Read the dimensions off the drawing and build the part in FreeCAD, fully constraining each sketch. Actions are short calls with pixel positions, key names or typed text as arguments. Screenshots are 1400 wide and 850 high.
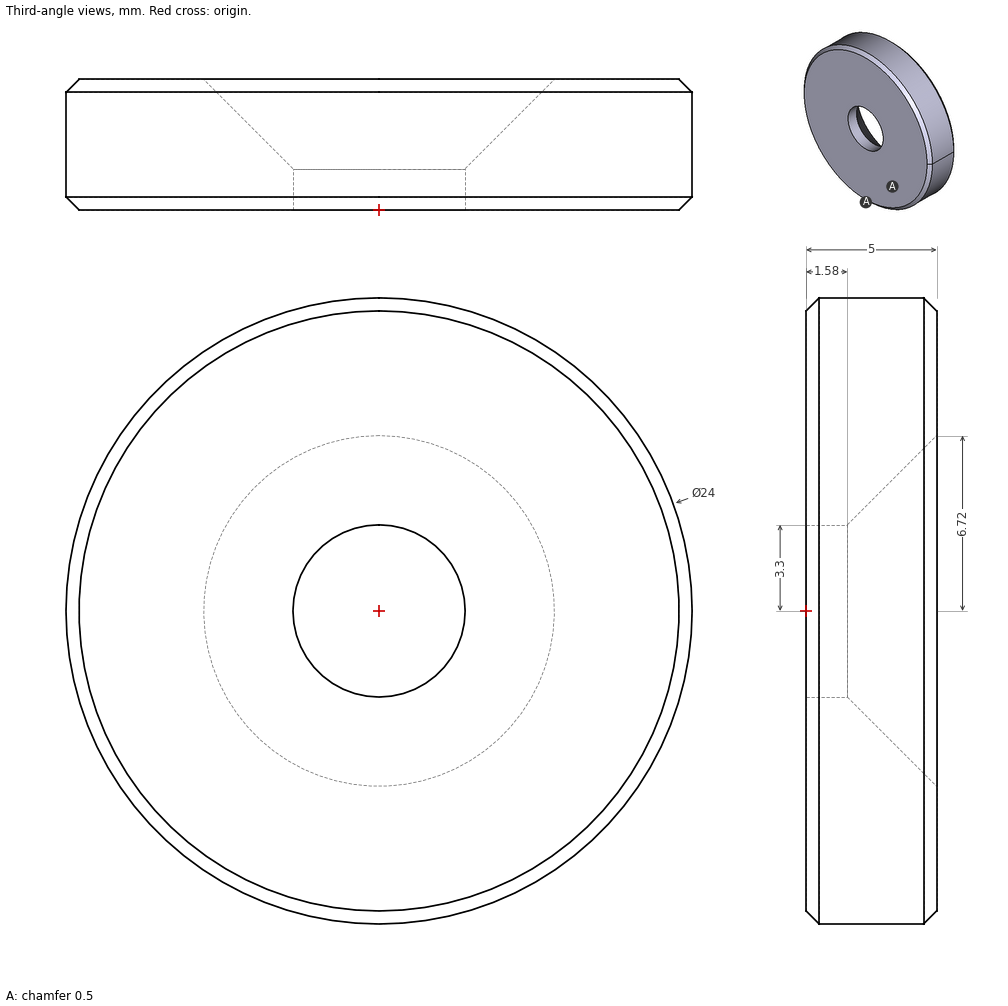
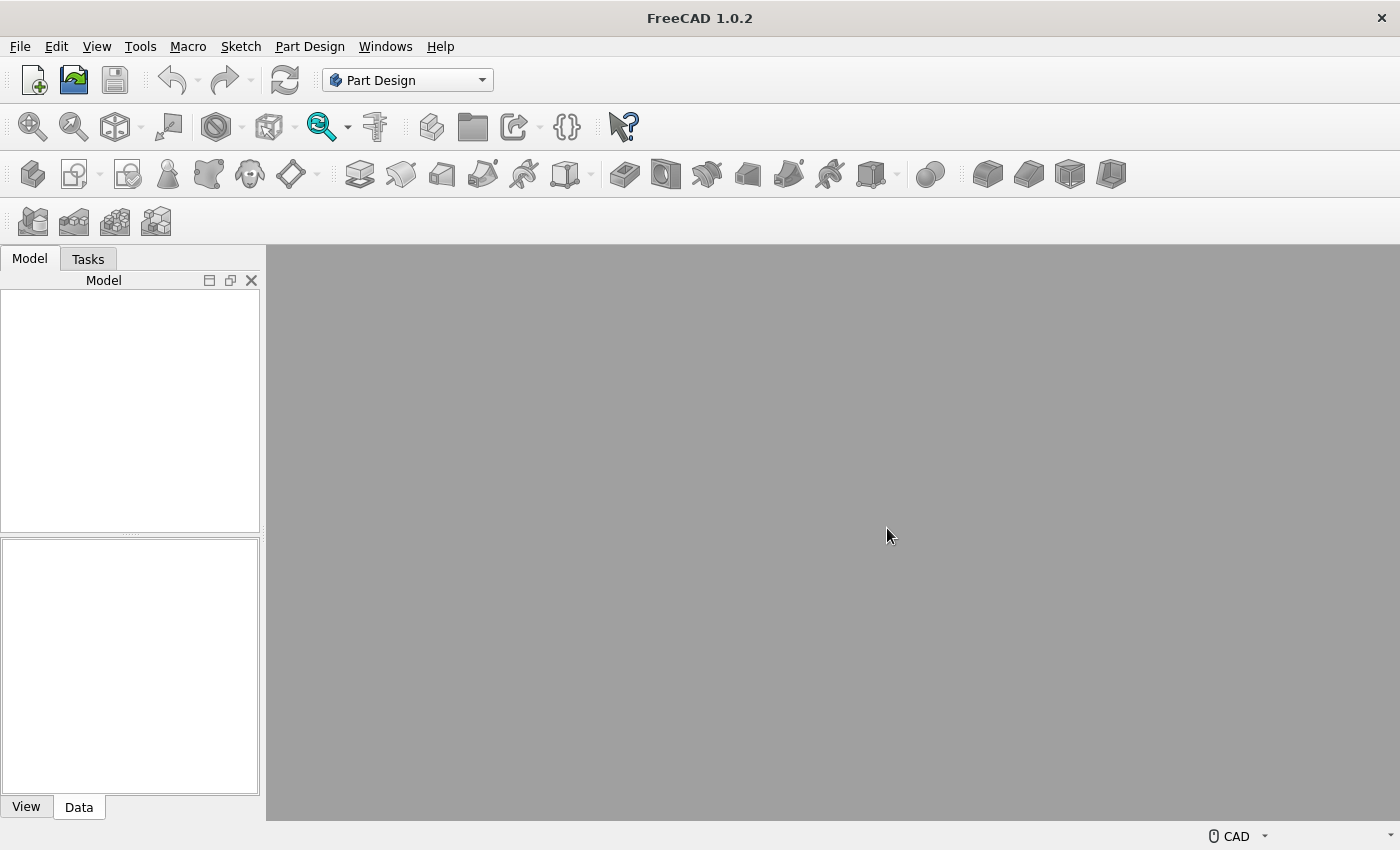
click(33, 80)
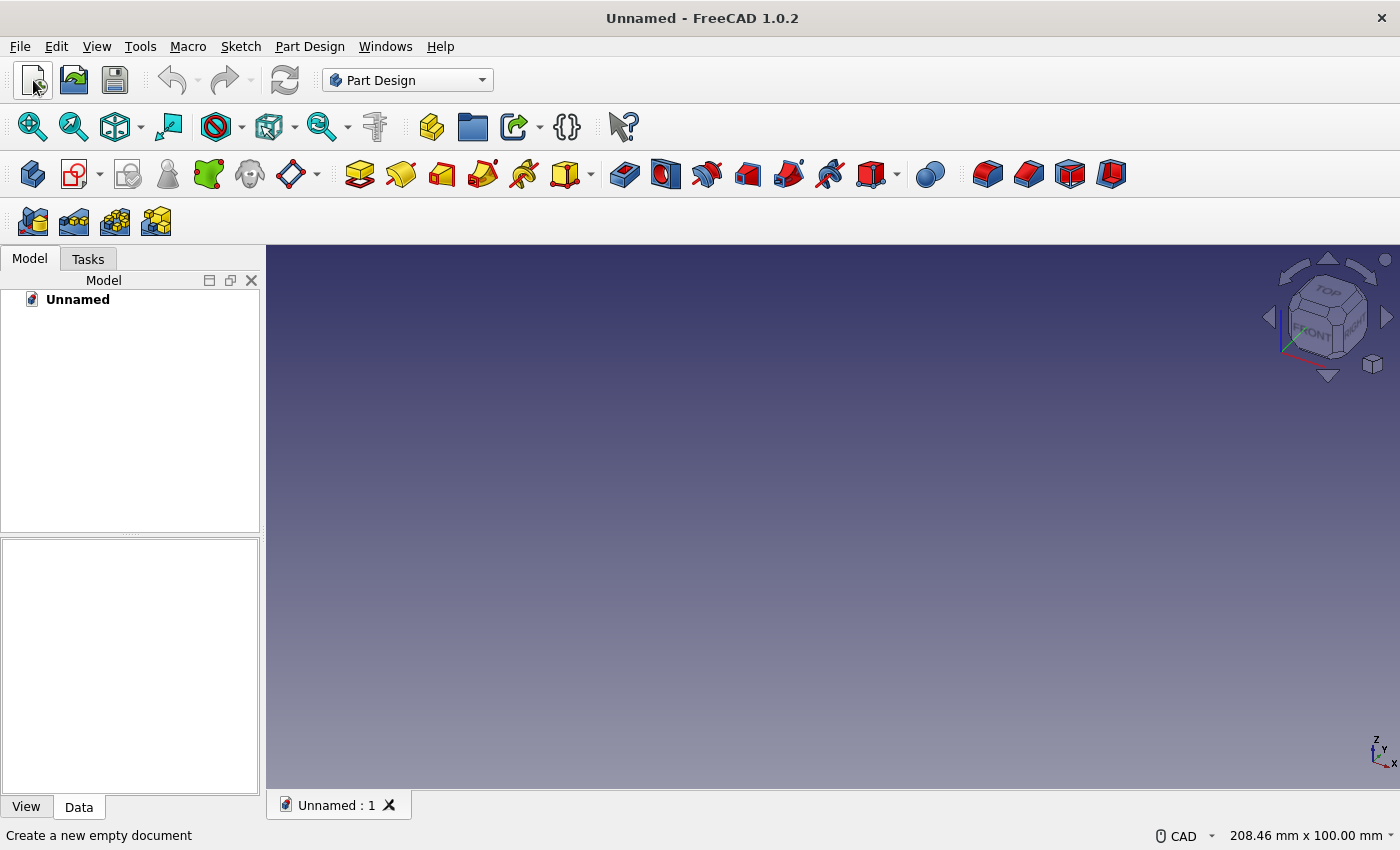
click(74, 174)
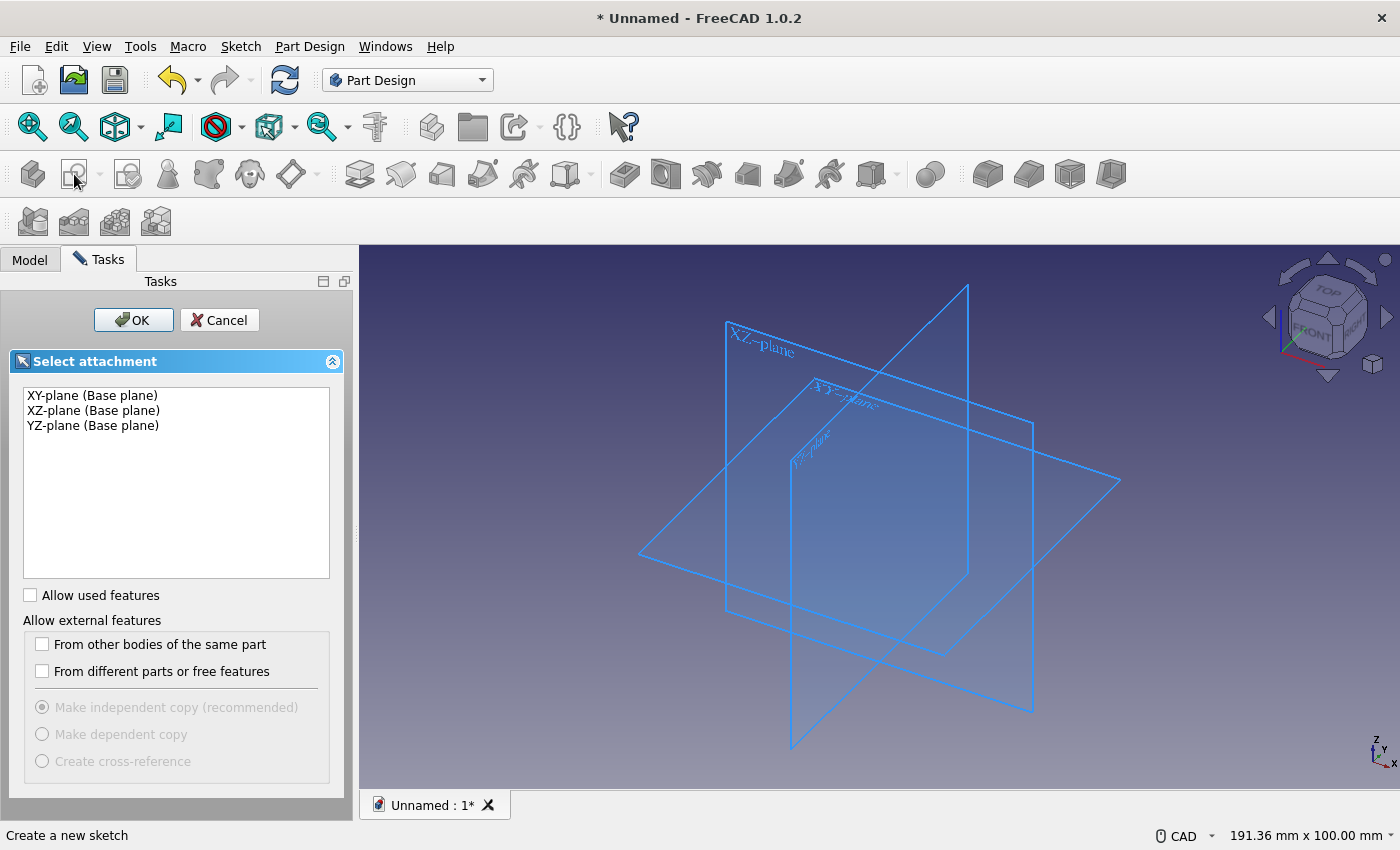
click(84, 410)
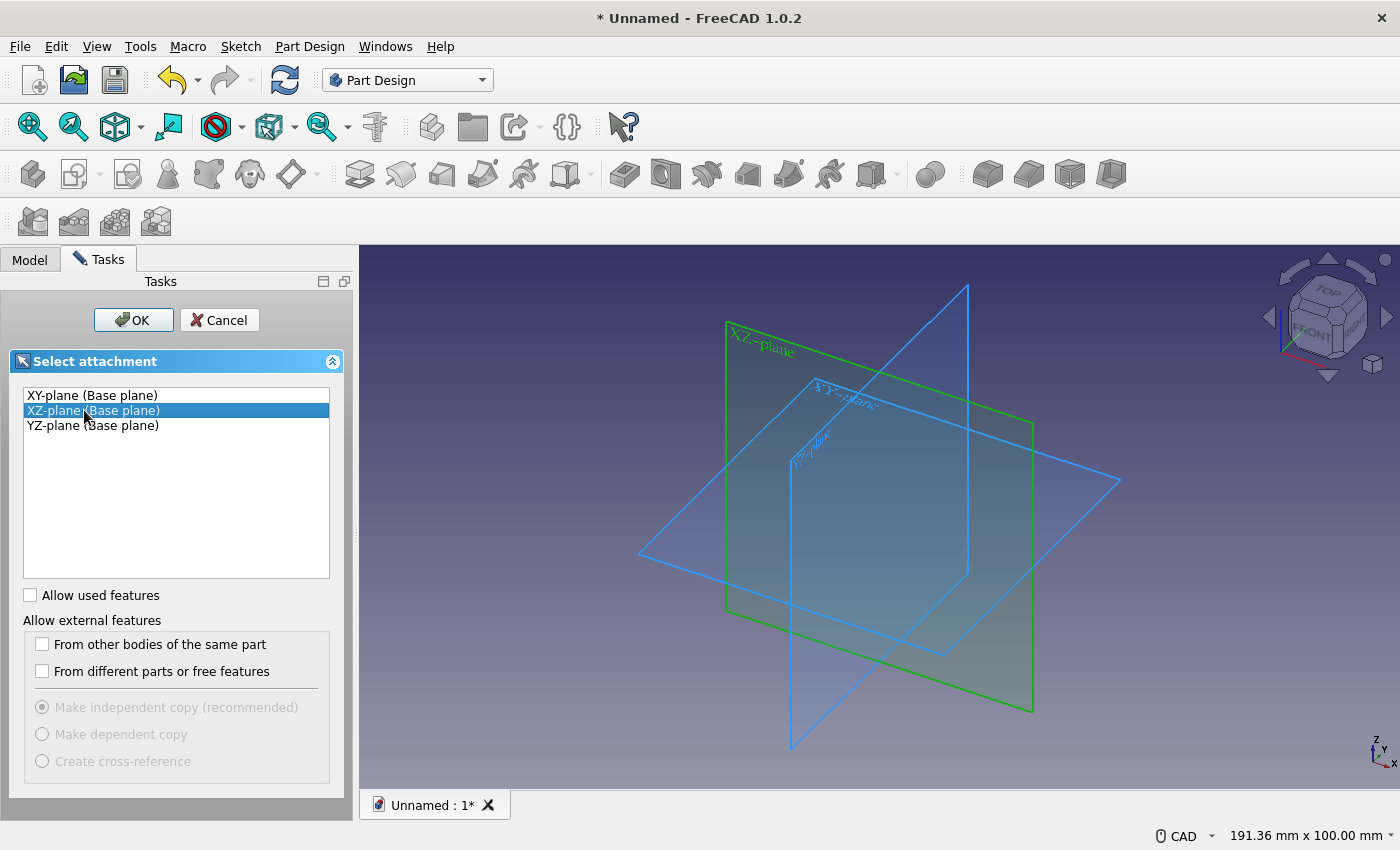
click(134, 320)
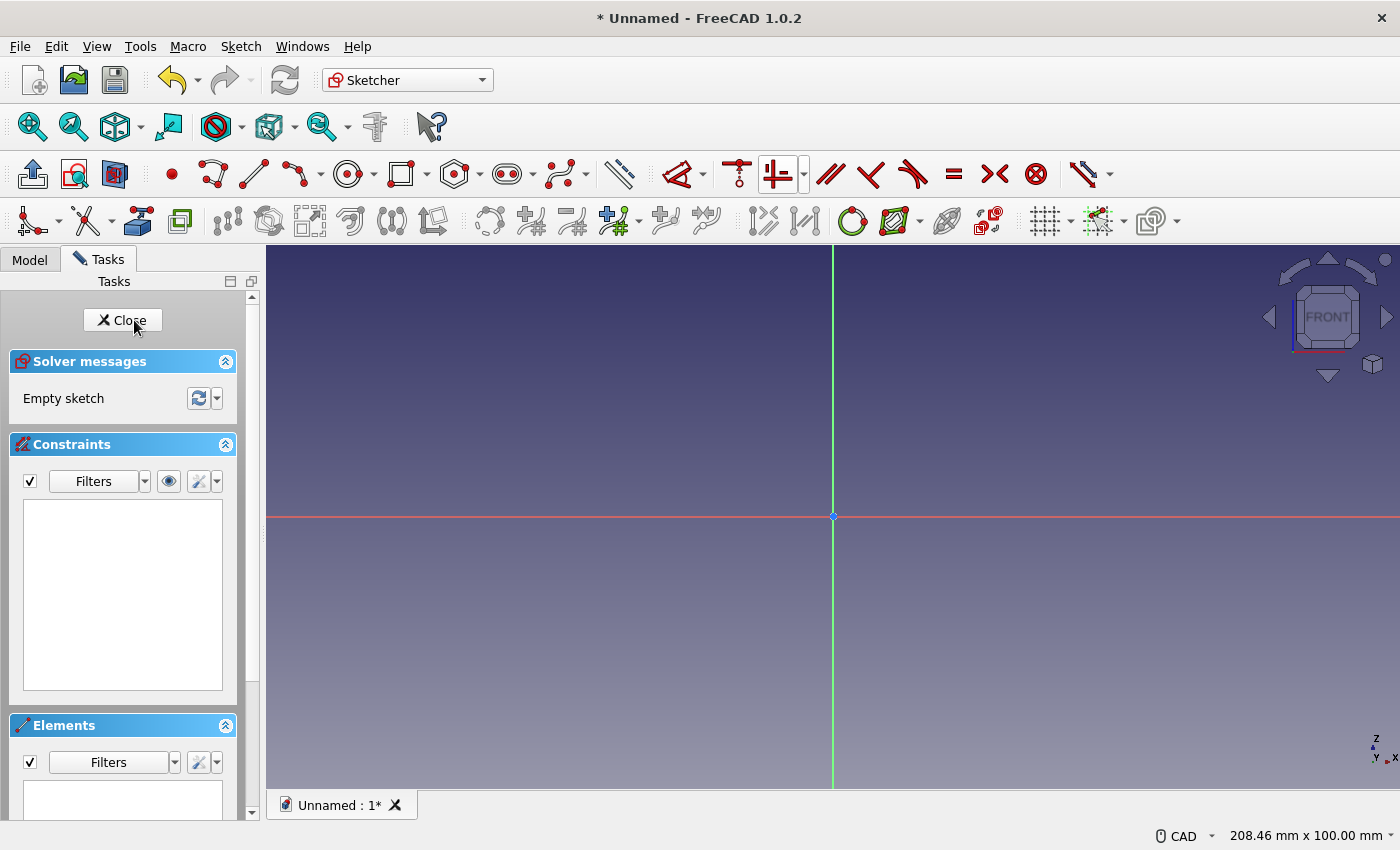
scroll(873, 517, up, 5)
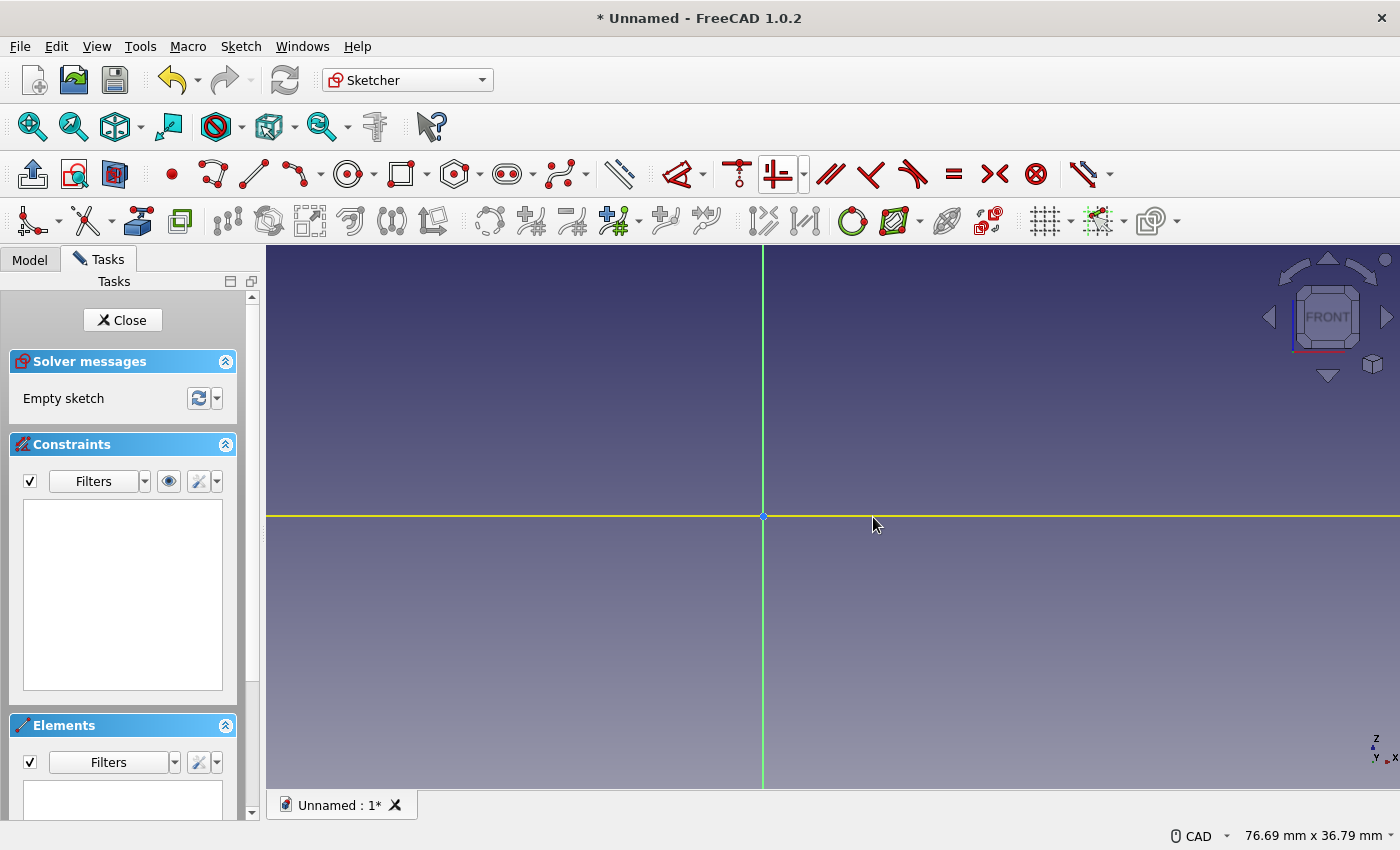
click(348, 174)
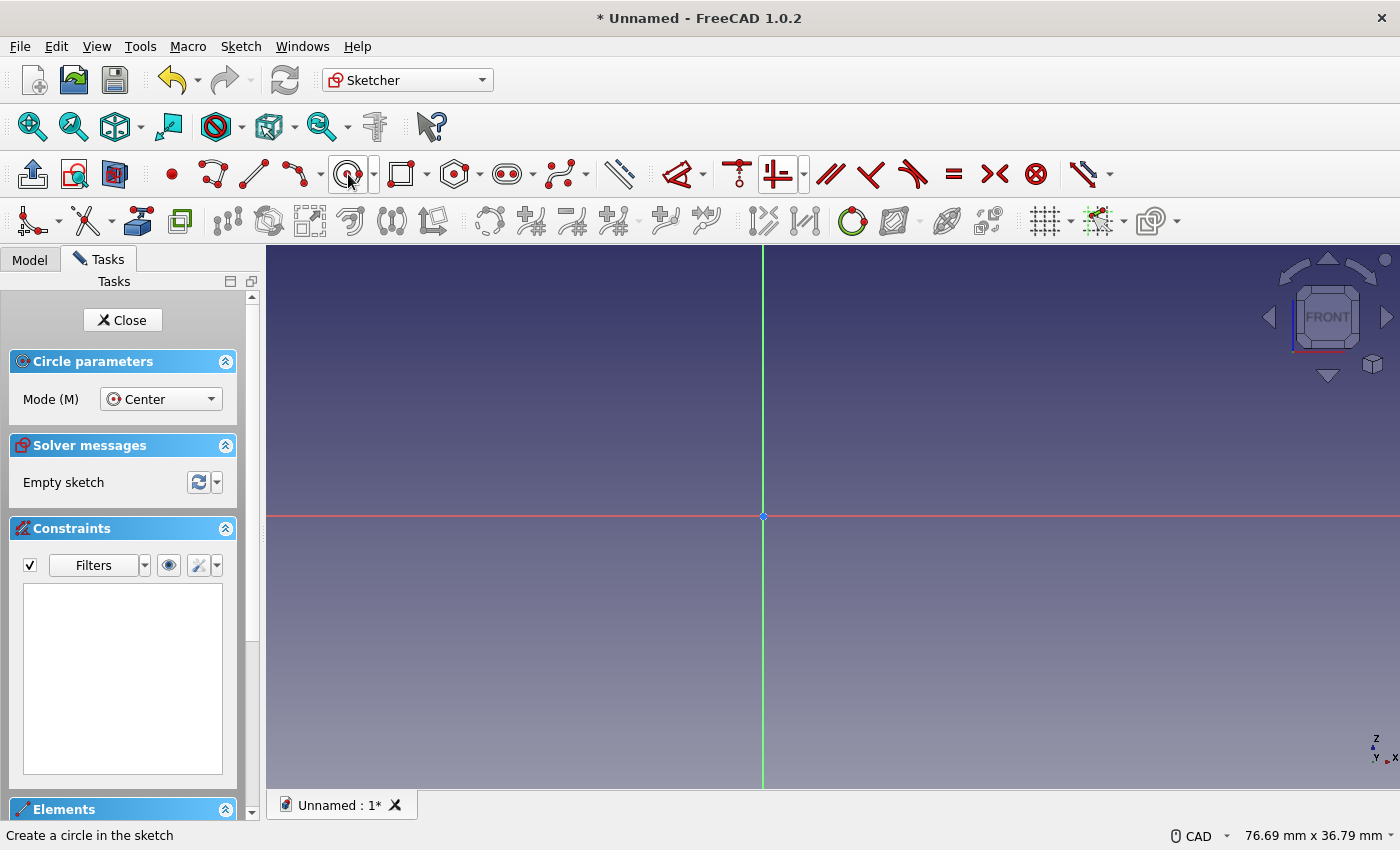
click(763, 516)
move(889, 391)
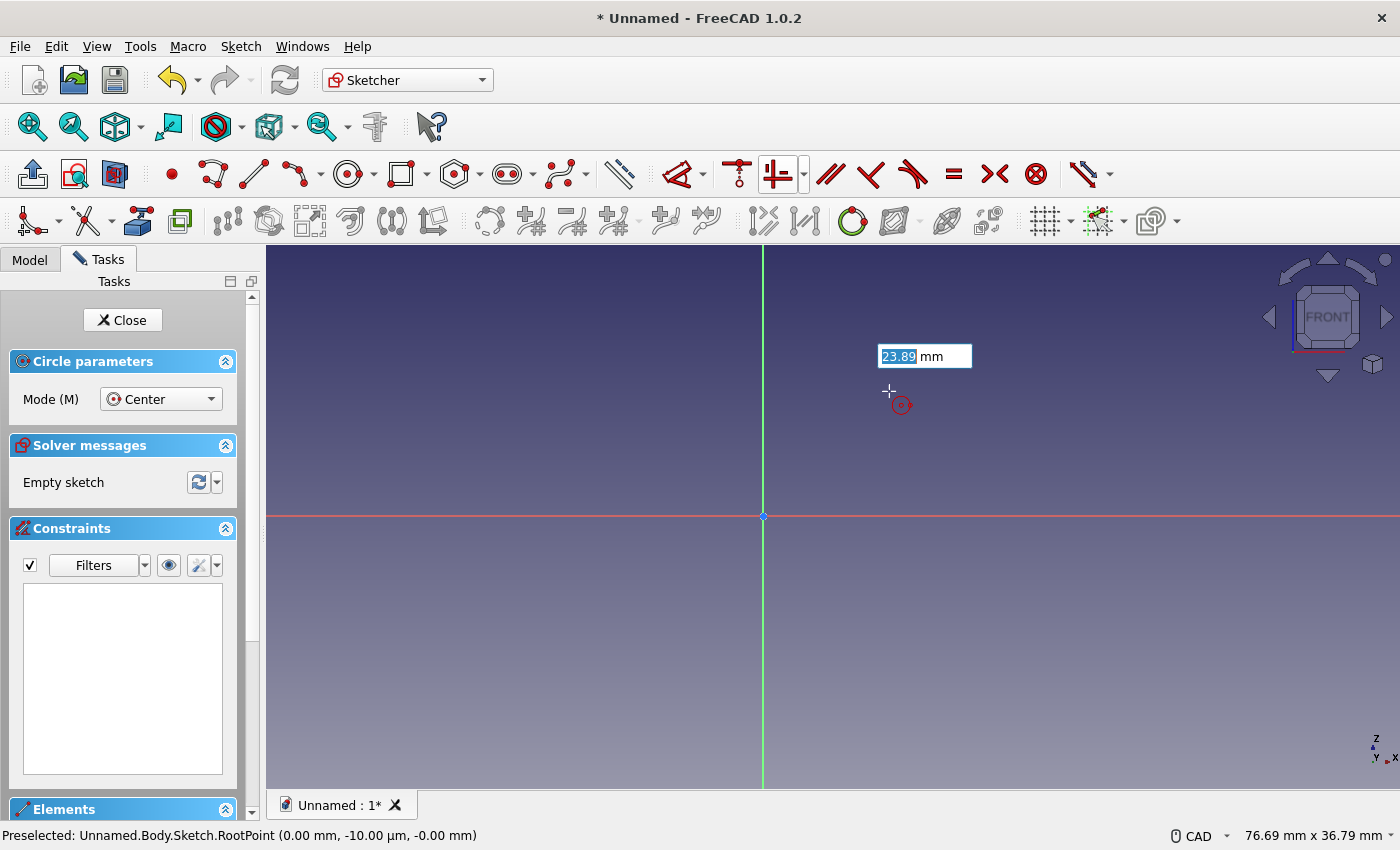
text(24)
key(Return)
key(Escape)